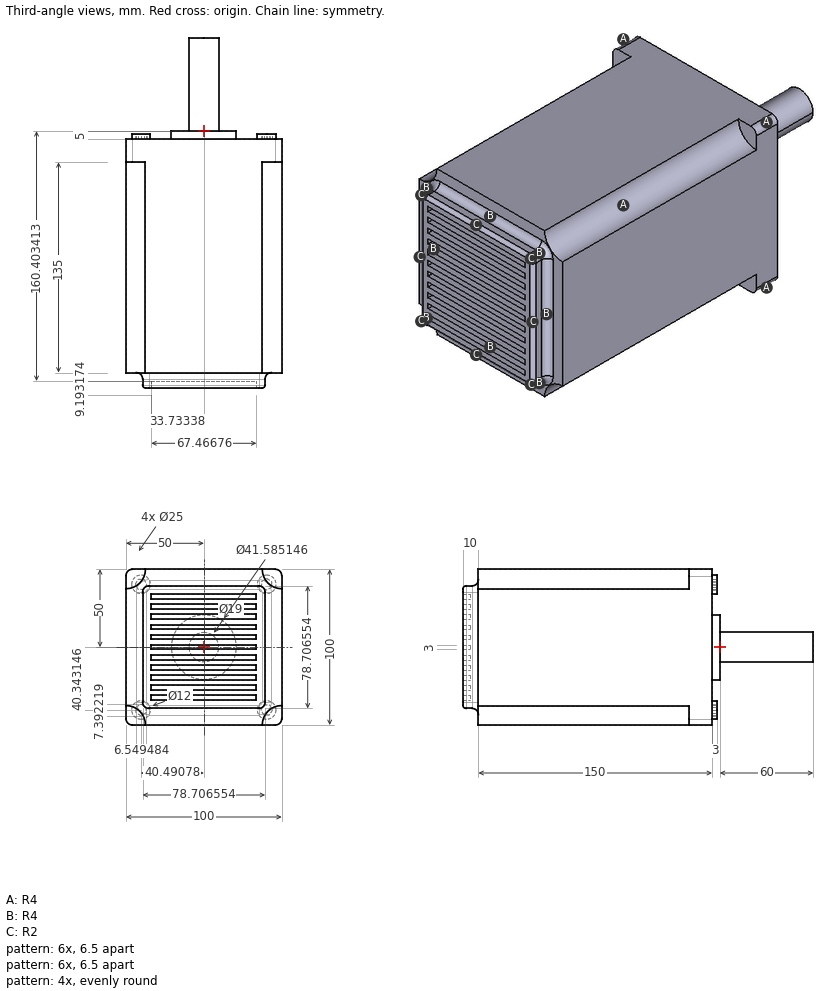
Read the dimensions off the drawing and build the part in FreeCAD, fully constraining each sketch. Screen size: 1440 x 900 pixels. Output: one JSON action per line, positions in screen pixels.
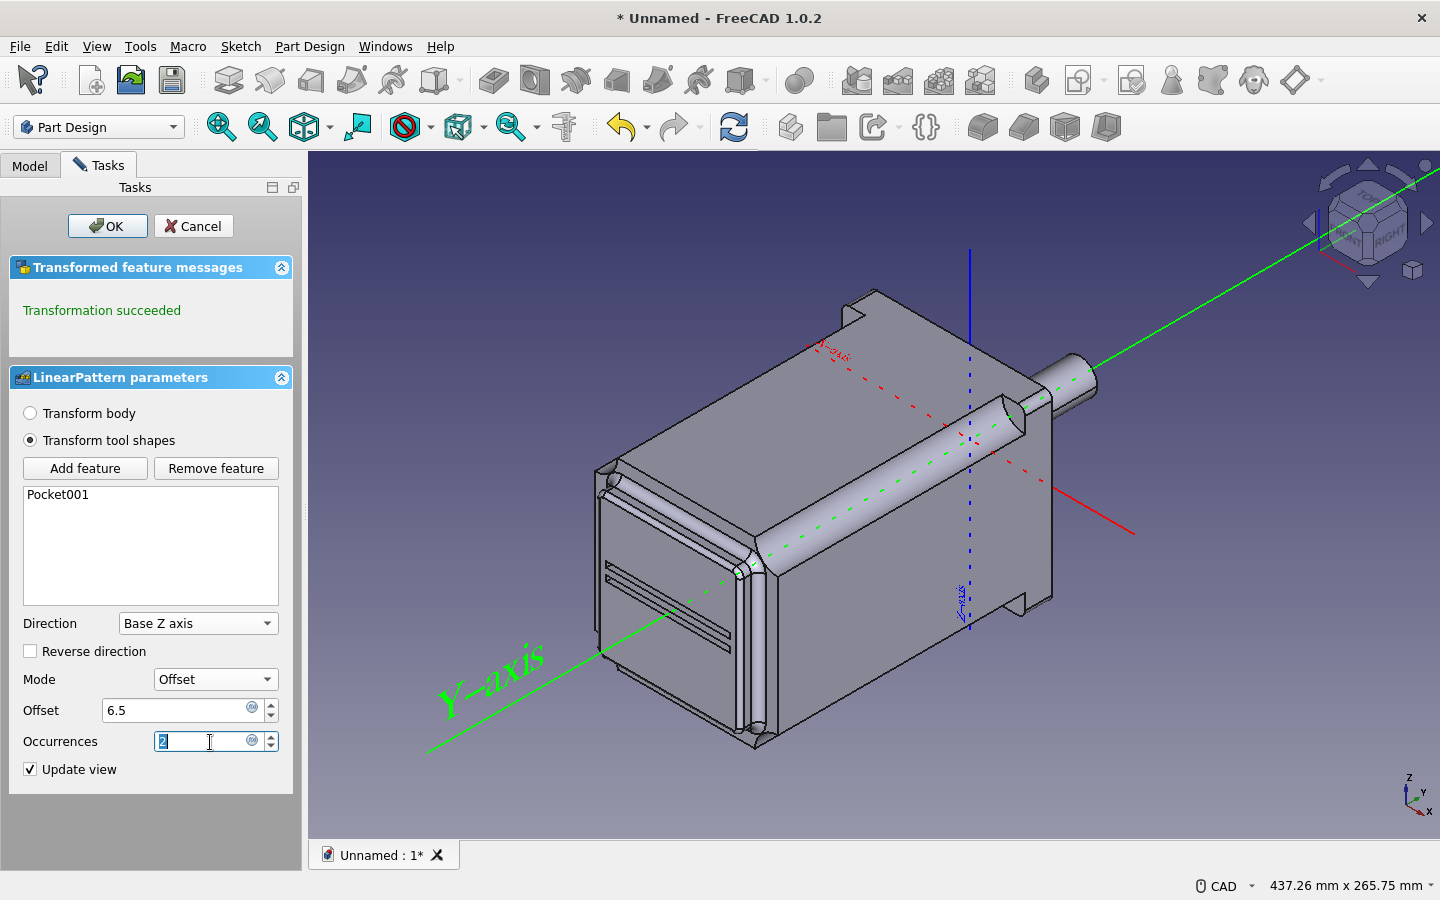
{"action": "type", "text": "6"}
{"action": "key", "text": "Tab"}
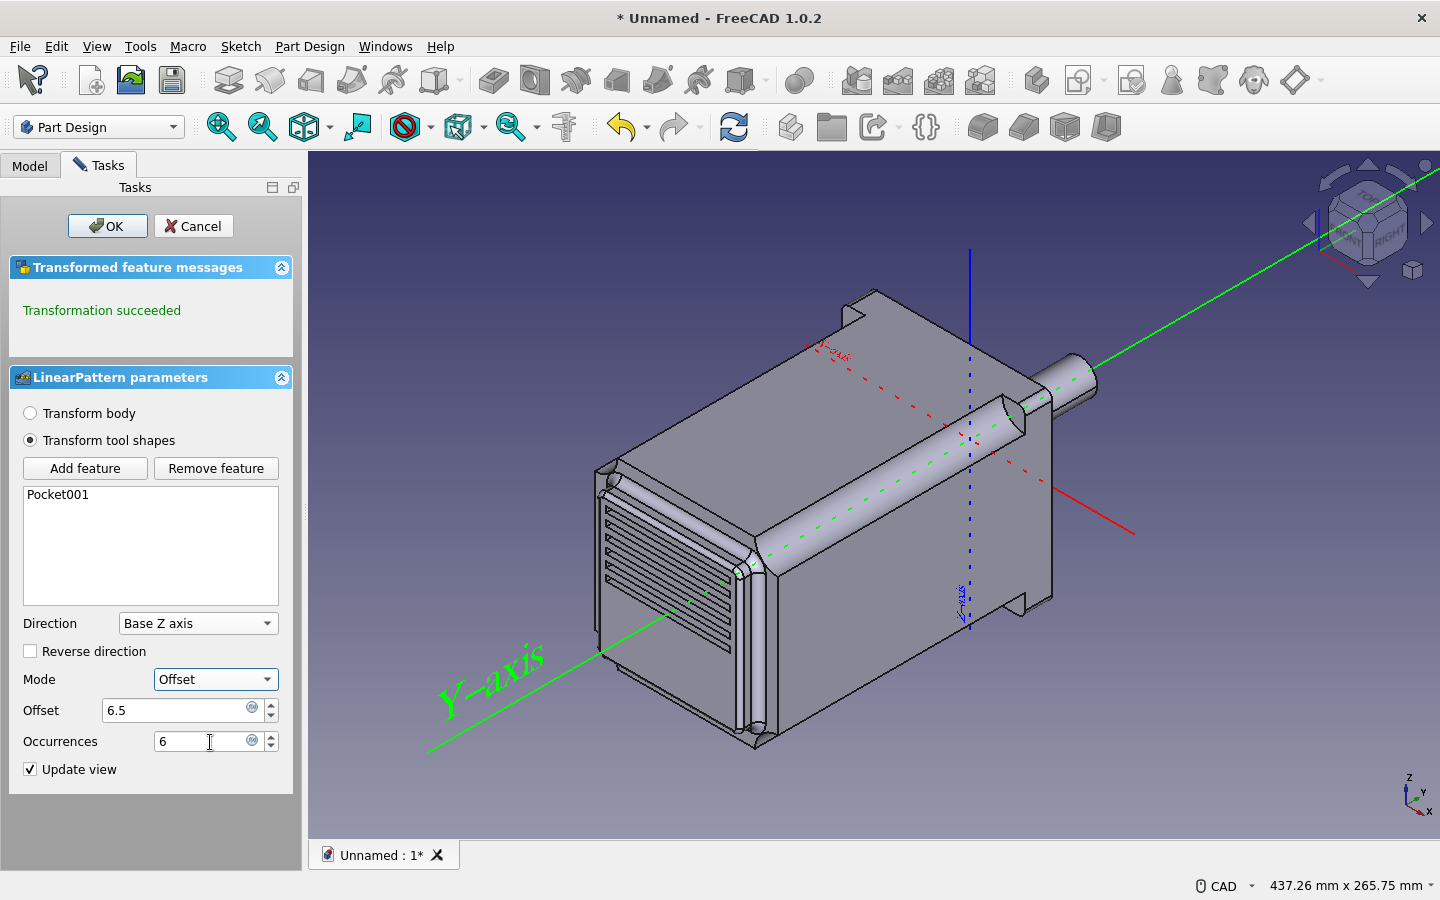
{"action": "left_click", "coordinate": [108, 226]}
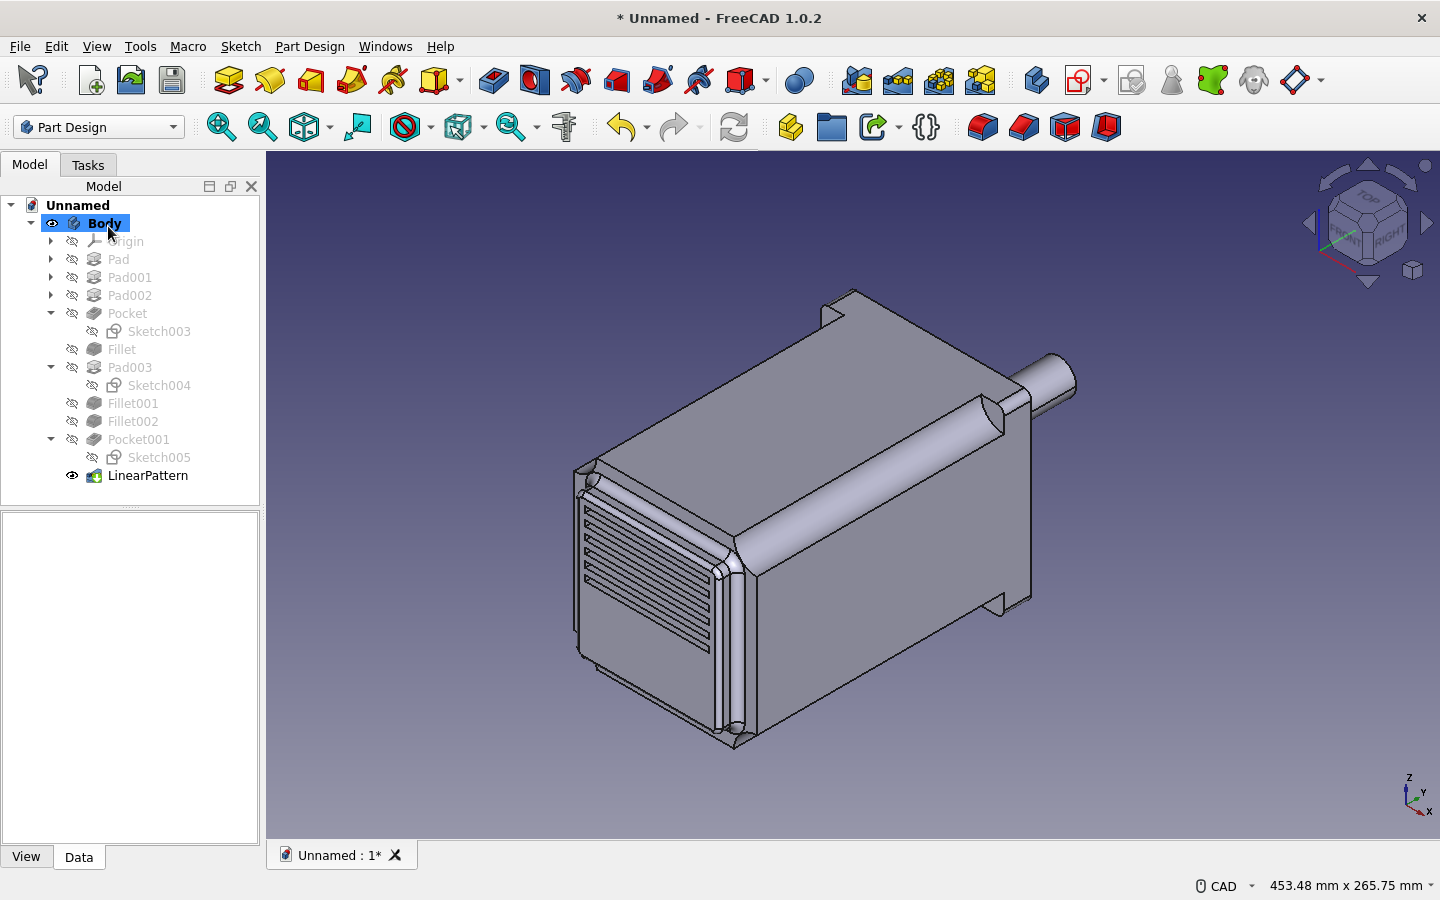
{"action": "left_click", "coordinate": [117, 439]}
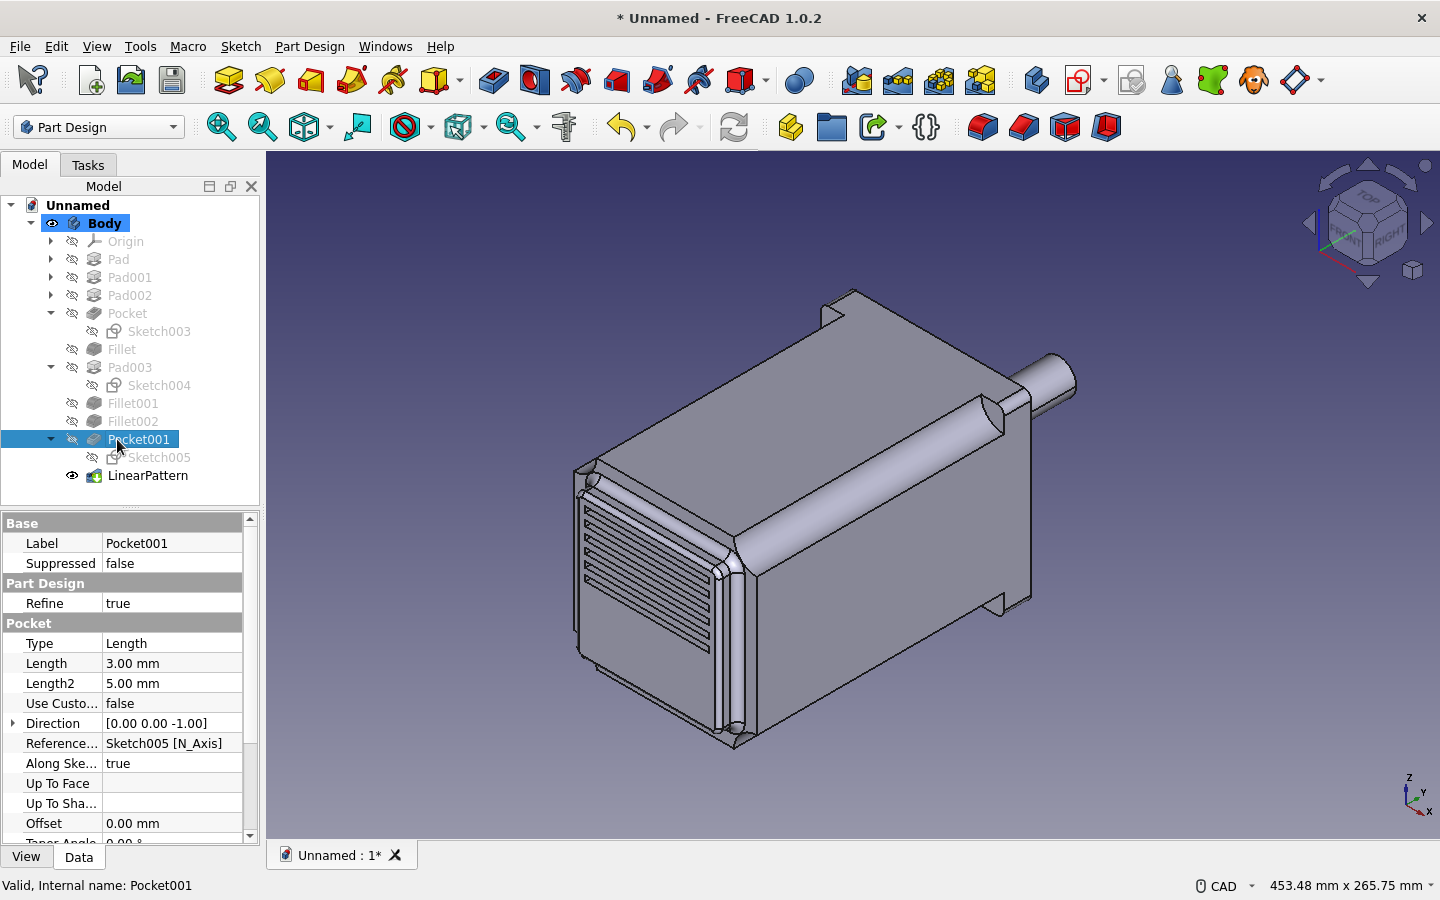
{"action": "left_click", "coordinate": [898, 80]}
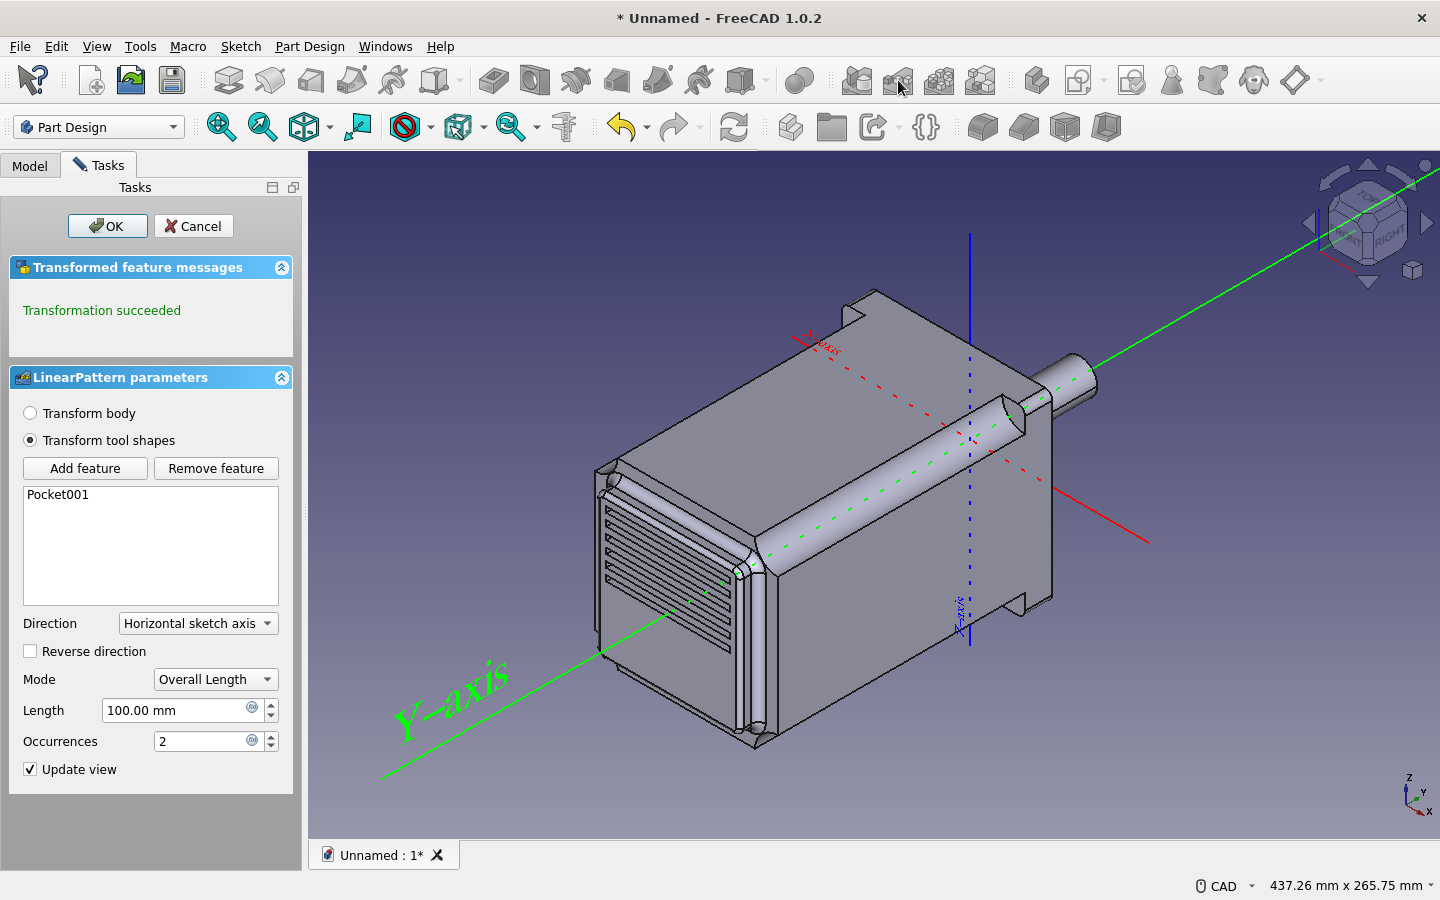
{"action": "left_click", "coordinate": [199, 624]}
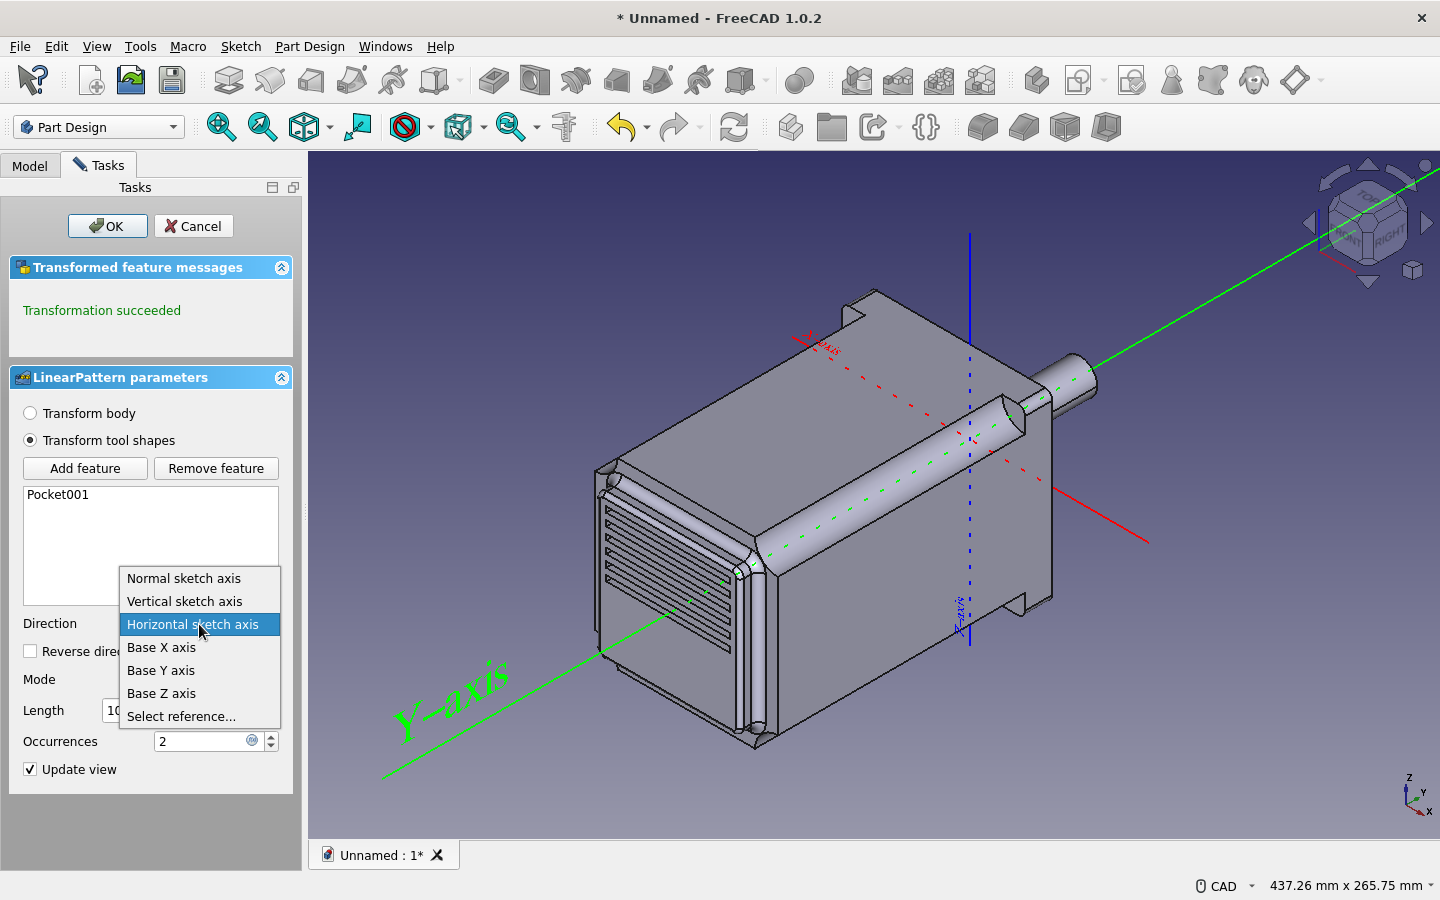
{"action": "left_click", "coordinate": [198, 694]}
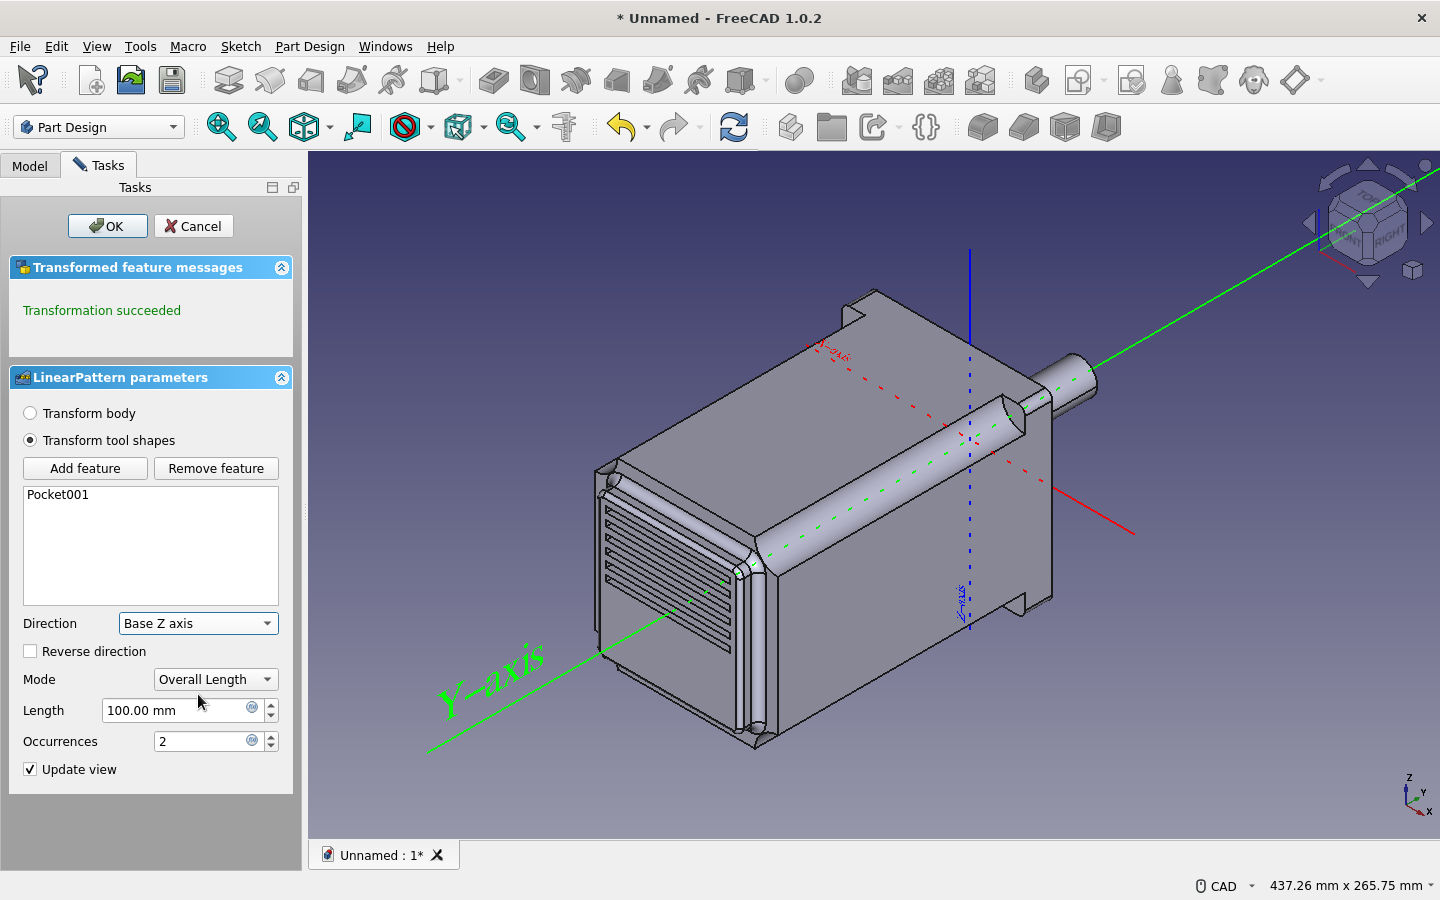
{"action": "left_click", "coordinate": [216, 680]}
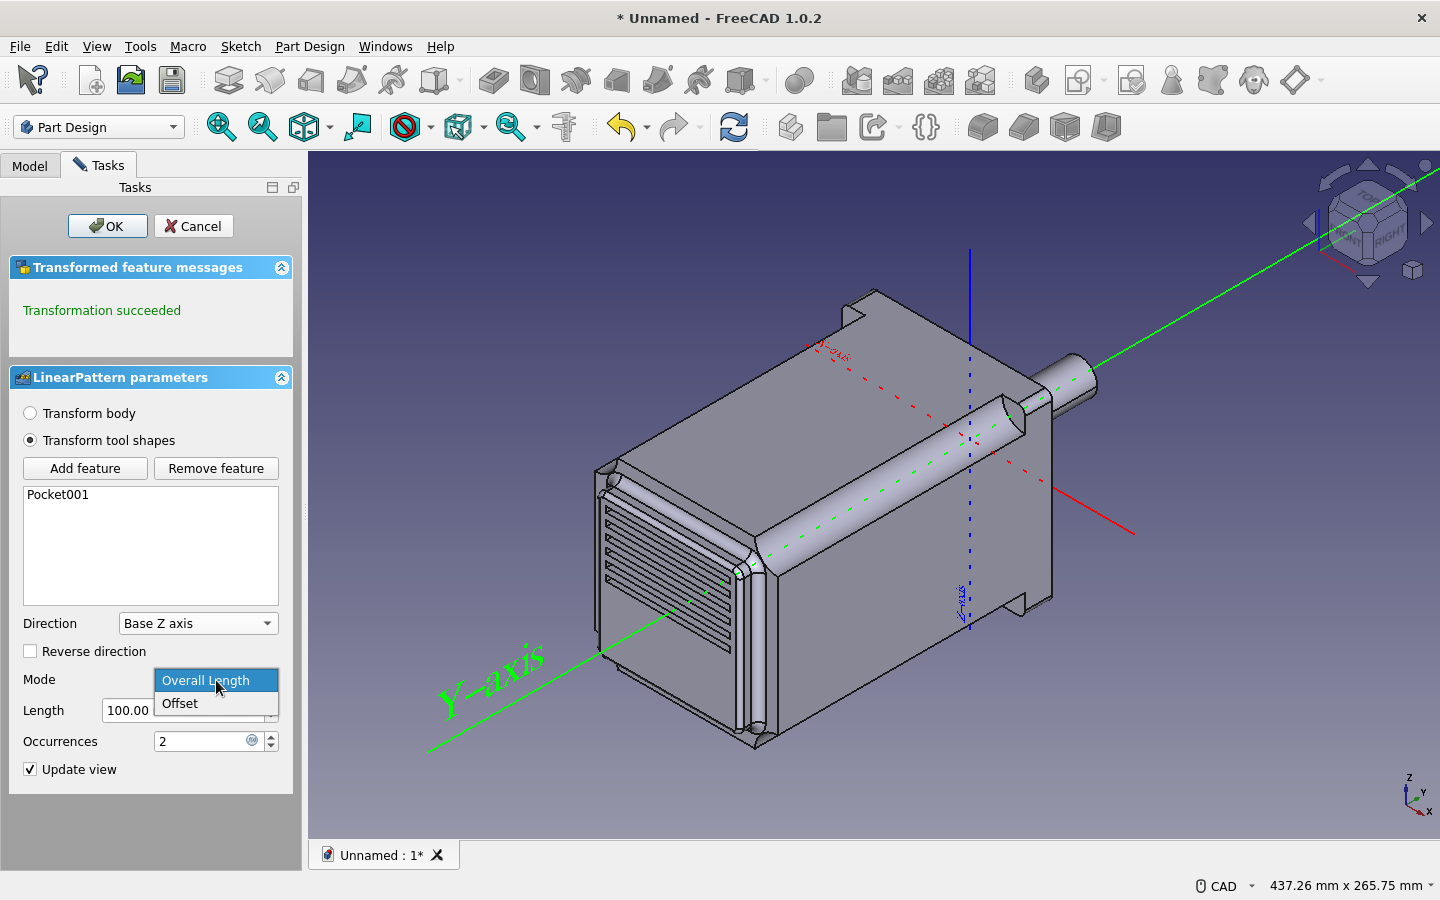
{"action": "left_click", "coordinate": [214, 704]}